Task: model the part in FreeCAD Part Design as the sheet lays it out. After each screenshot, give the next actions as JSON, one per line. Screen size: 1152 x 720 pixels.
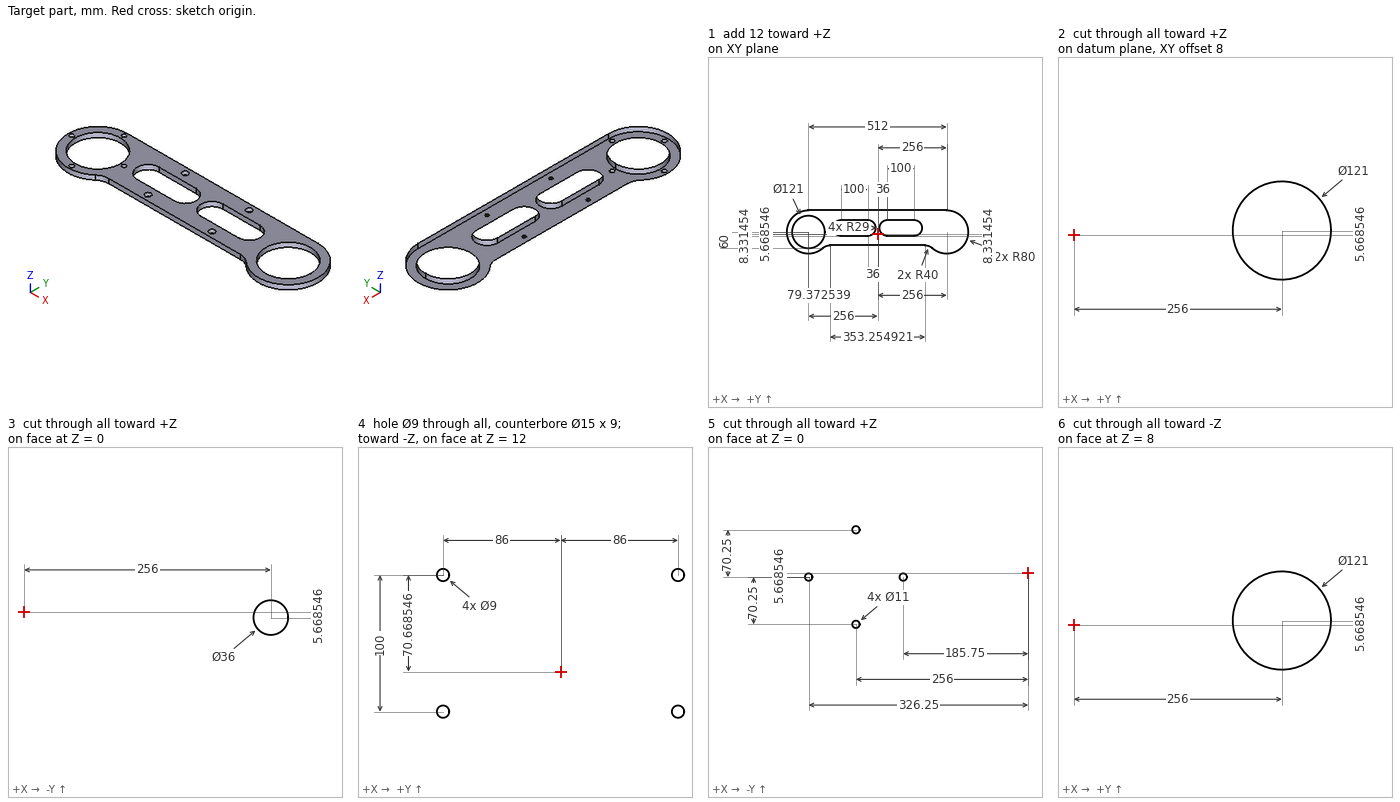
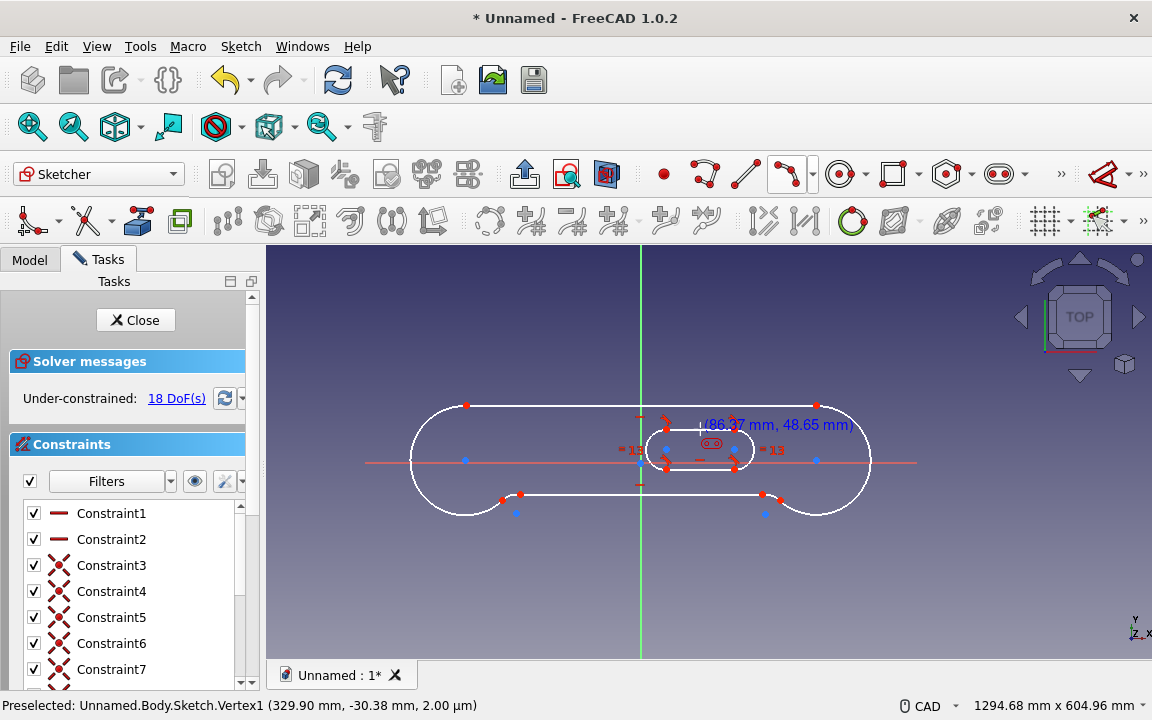
{"action": "left_click", "coordinate": [548, 449]}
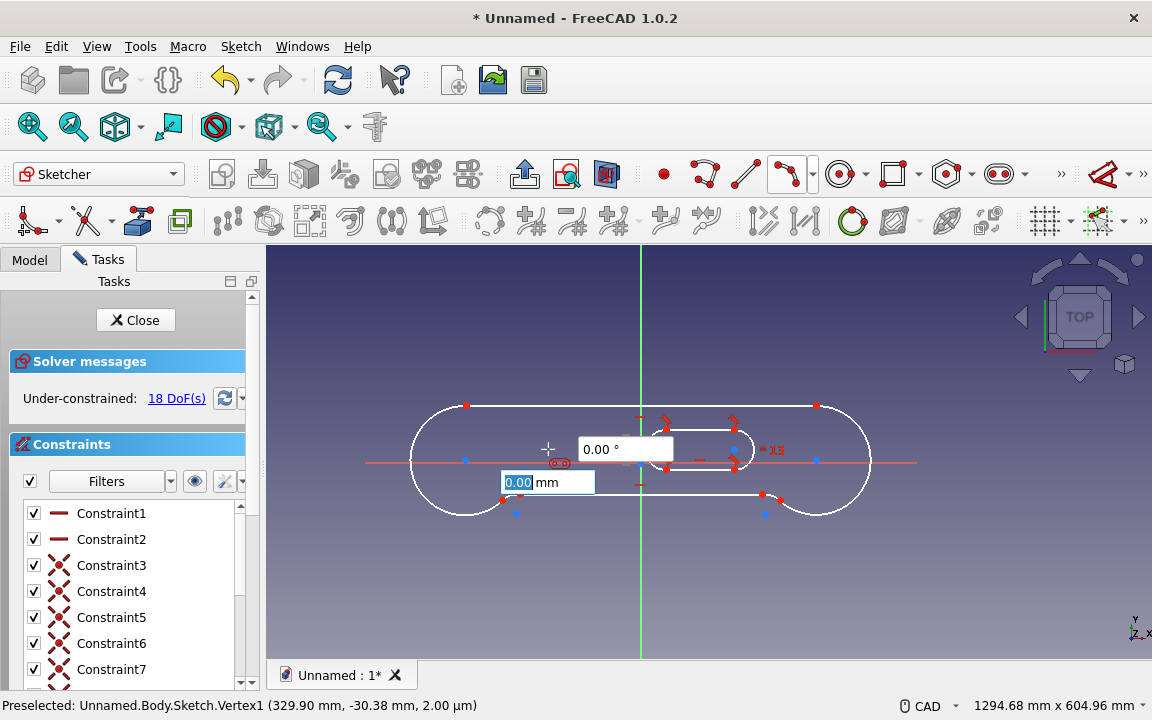
{"action": "left_click", "coordinate": [616, 449]}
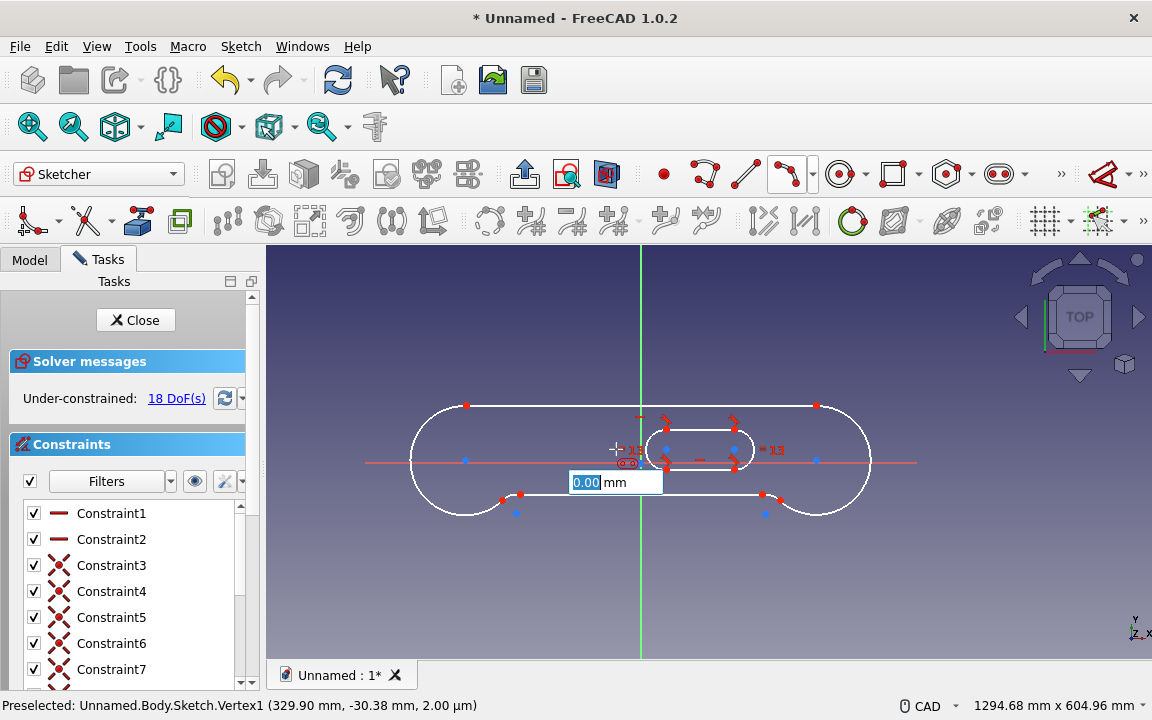
{"action": "left_click", "coordinate": [582, 429]}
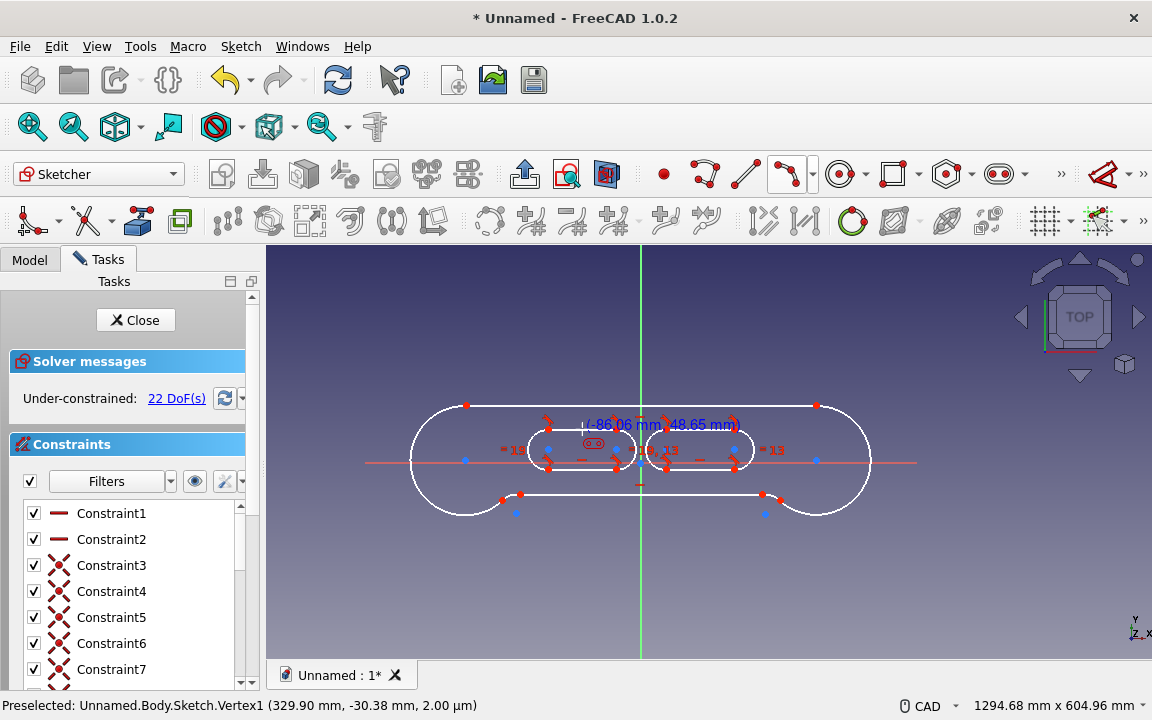
{"action": "left_click", "coordinate": [840, 174]}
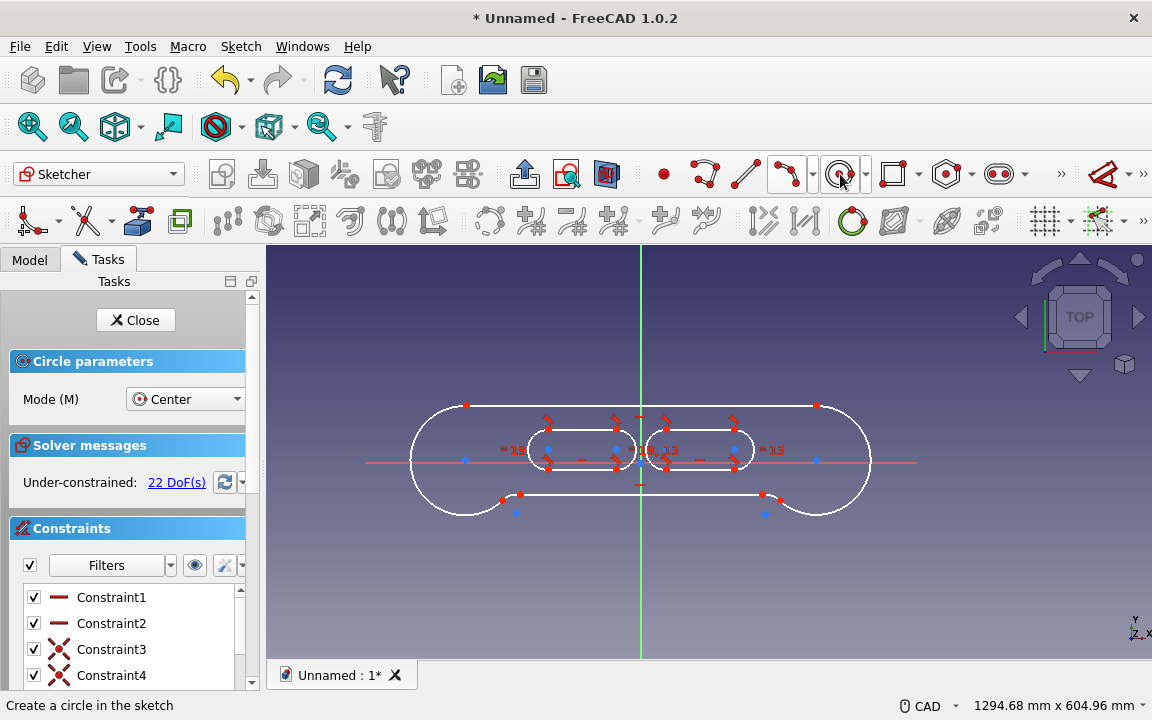
{"action": "scroll", "coordinate": [466, 459], "scroll_direction": "up", "scroll_amount": 8}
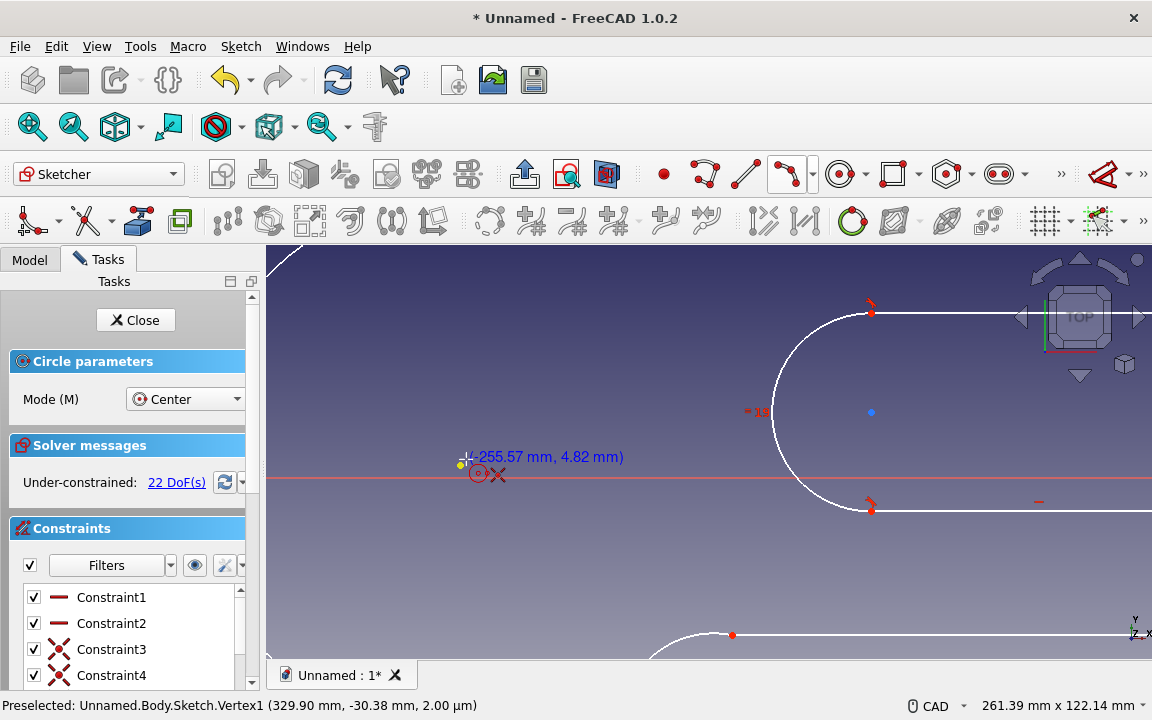
{"action": "left_click", "coordinate": [464, 459]}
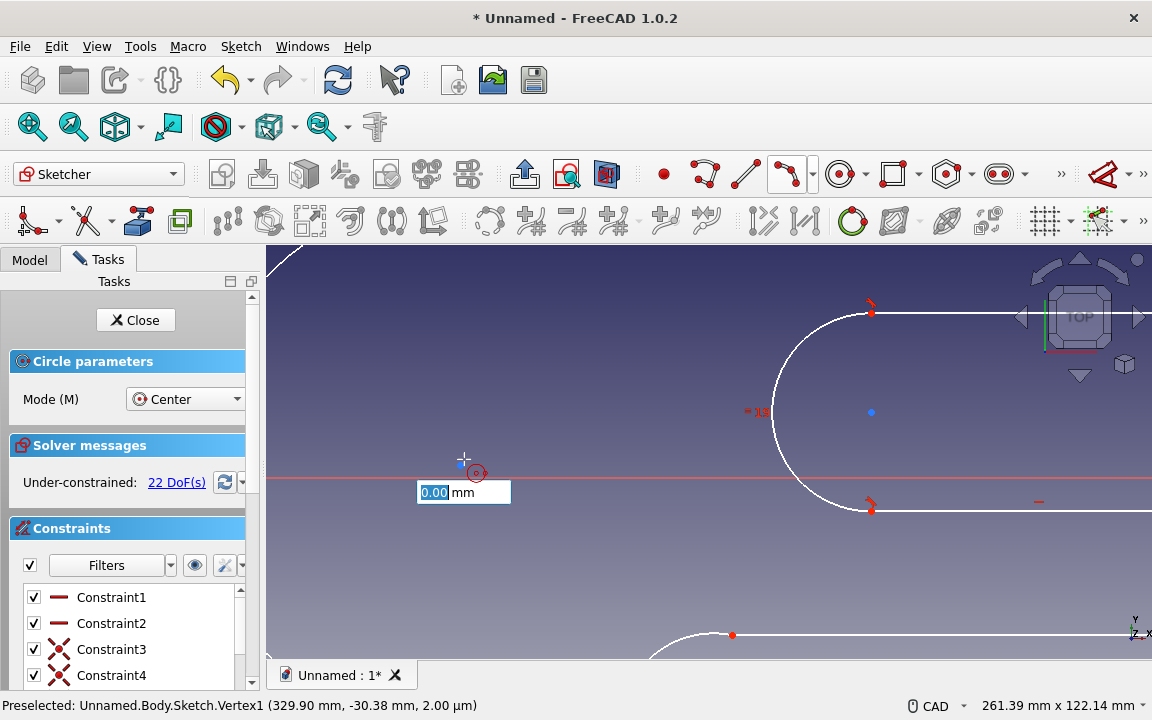
{"action": "scroll", "coordinate": [466, 459], "scroll_direction": "down", "scroll_amount": 8}
{"action": "mouse_move", "coordinate": [495, 430]}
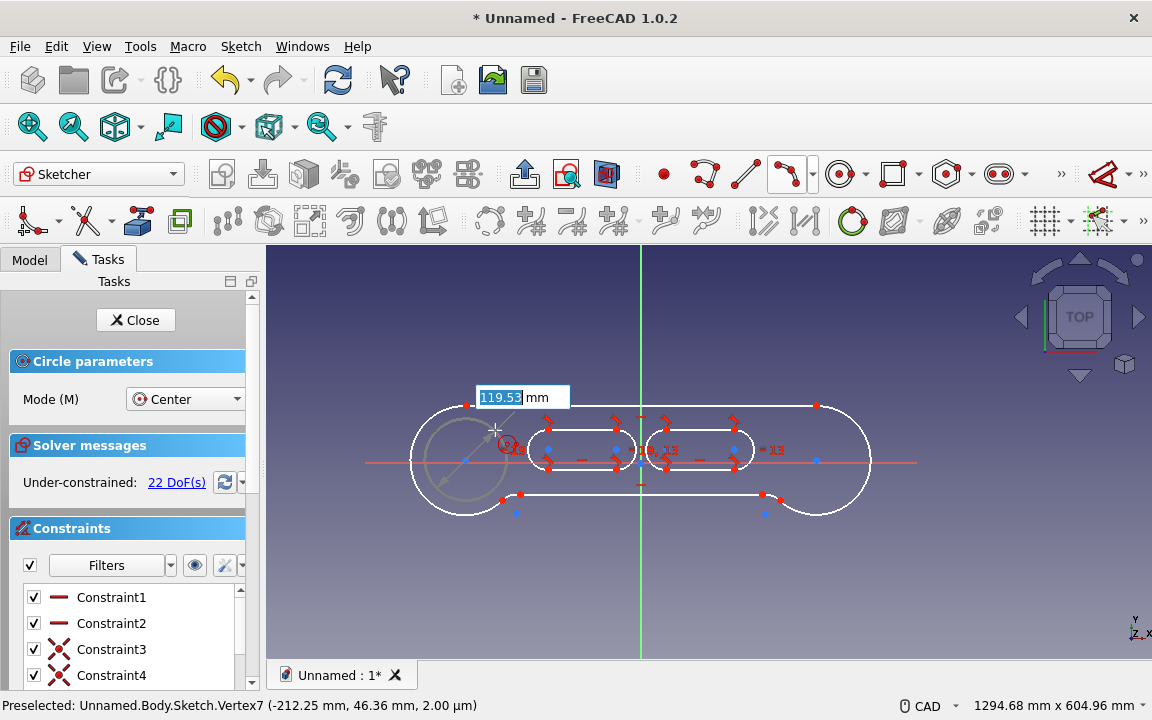
{"action": "type", "text": "121"}
{"action": "key", "text": "Return"}
{"action": "key", "text": "Escape"}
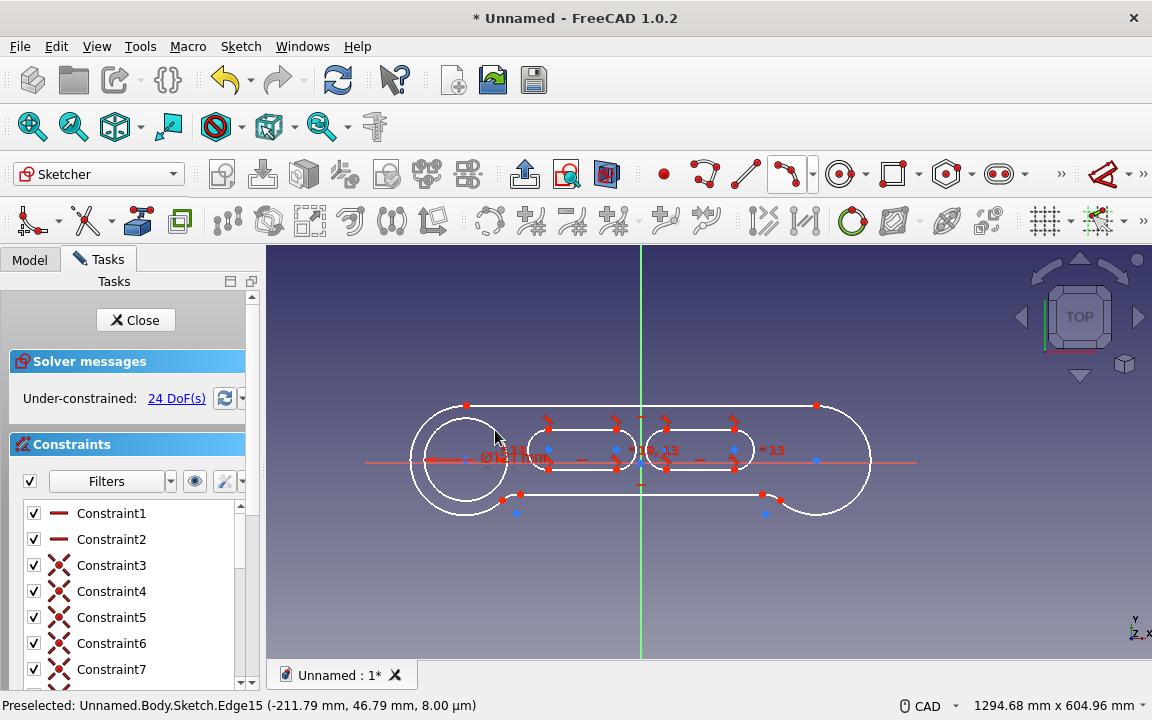
{"action": "left_click", "coordinate": [415, 438]}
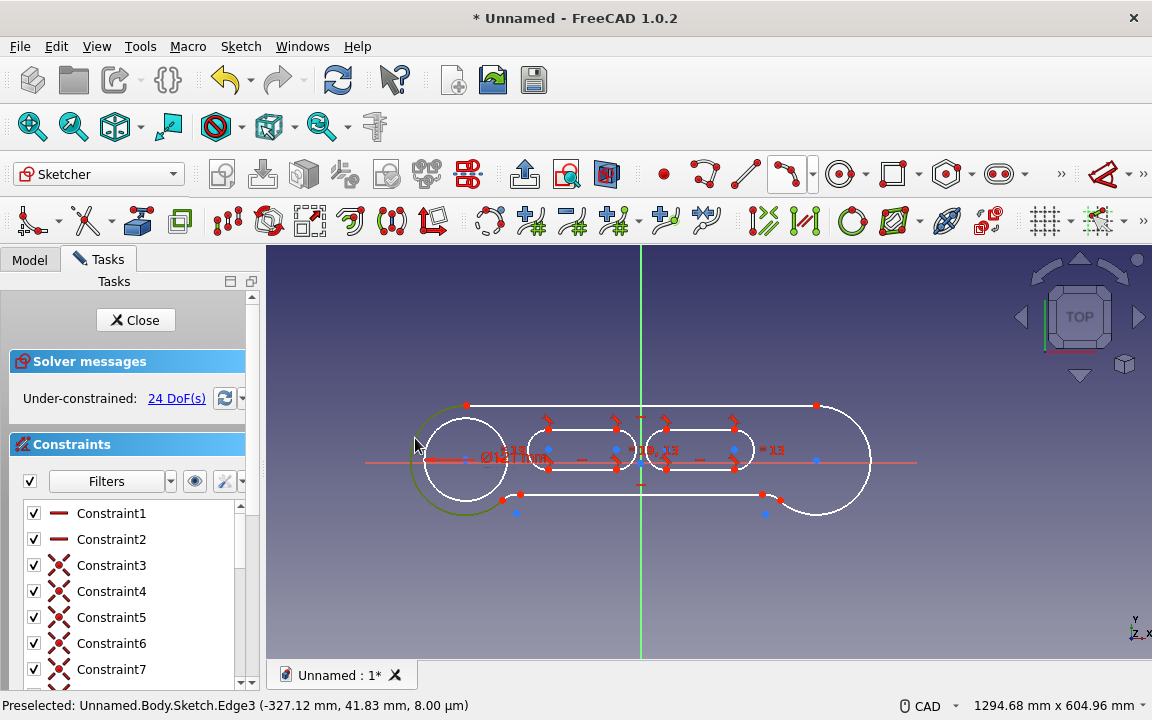
{"action": "scroll", "coordinate": [510, 496], "scroll_direction": "up", "scroll_amount": 2}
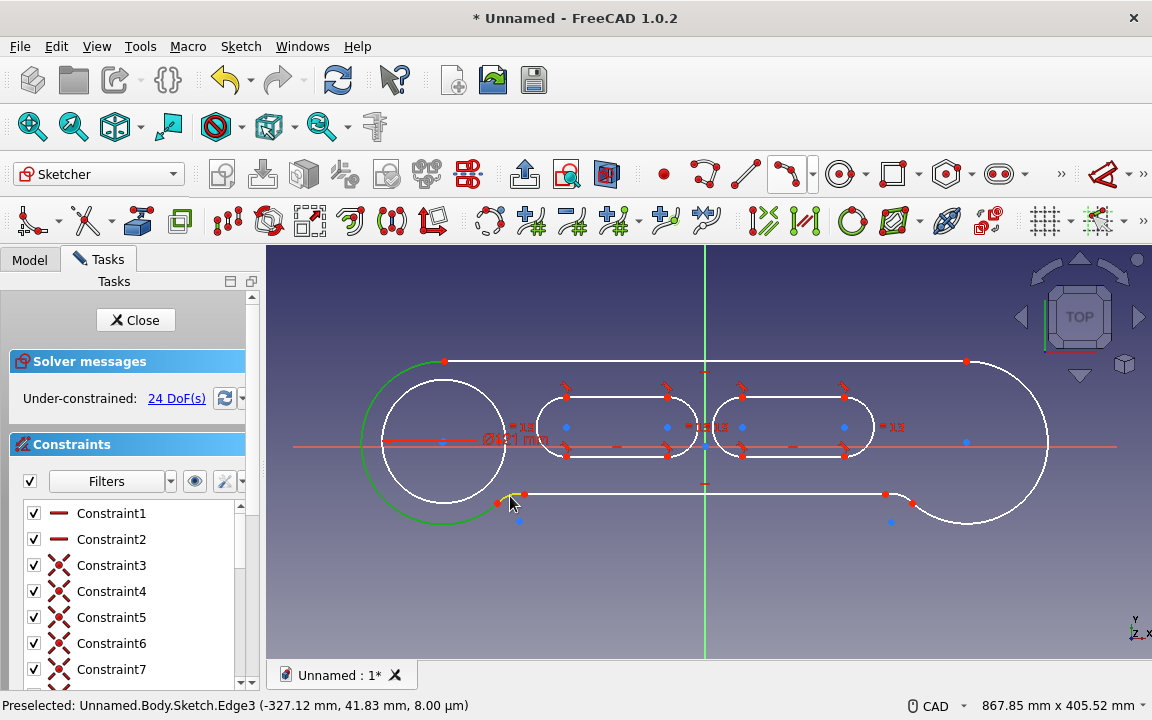
{"action": "left_click", "coordinate": [510, 495]}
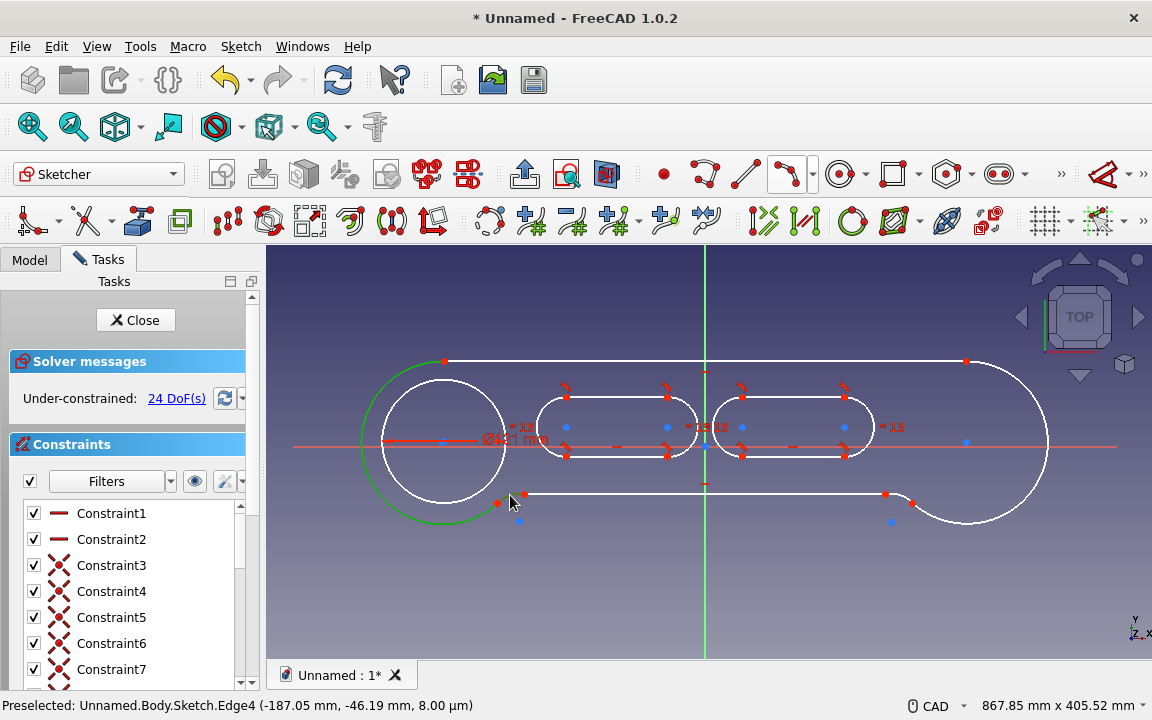
{"action": "key", "text": "t"}